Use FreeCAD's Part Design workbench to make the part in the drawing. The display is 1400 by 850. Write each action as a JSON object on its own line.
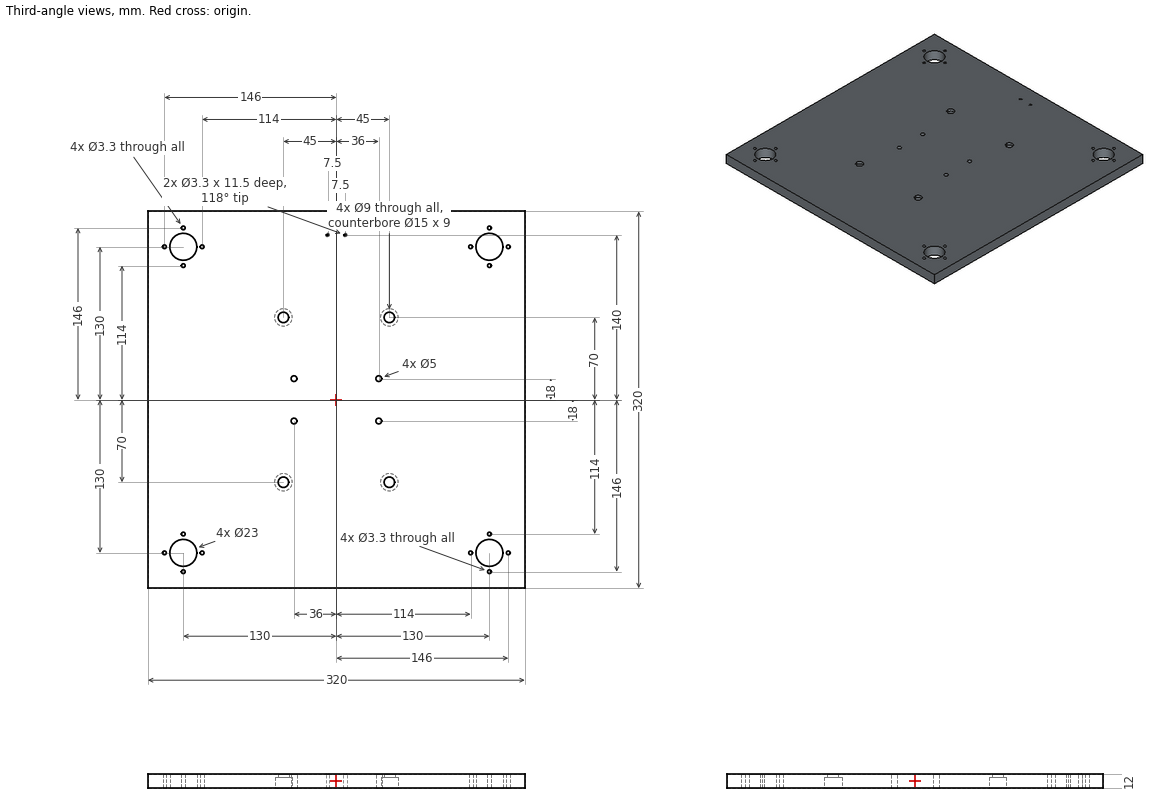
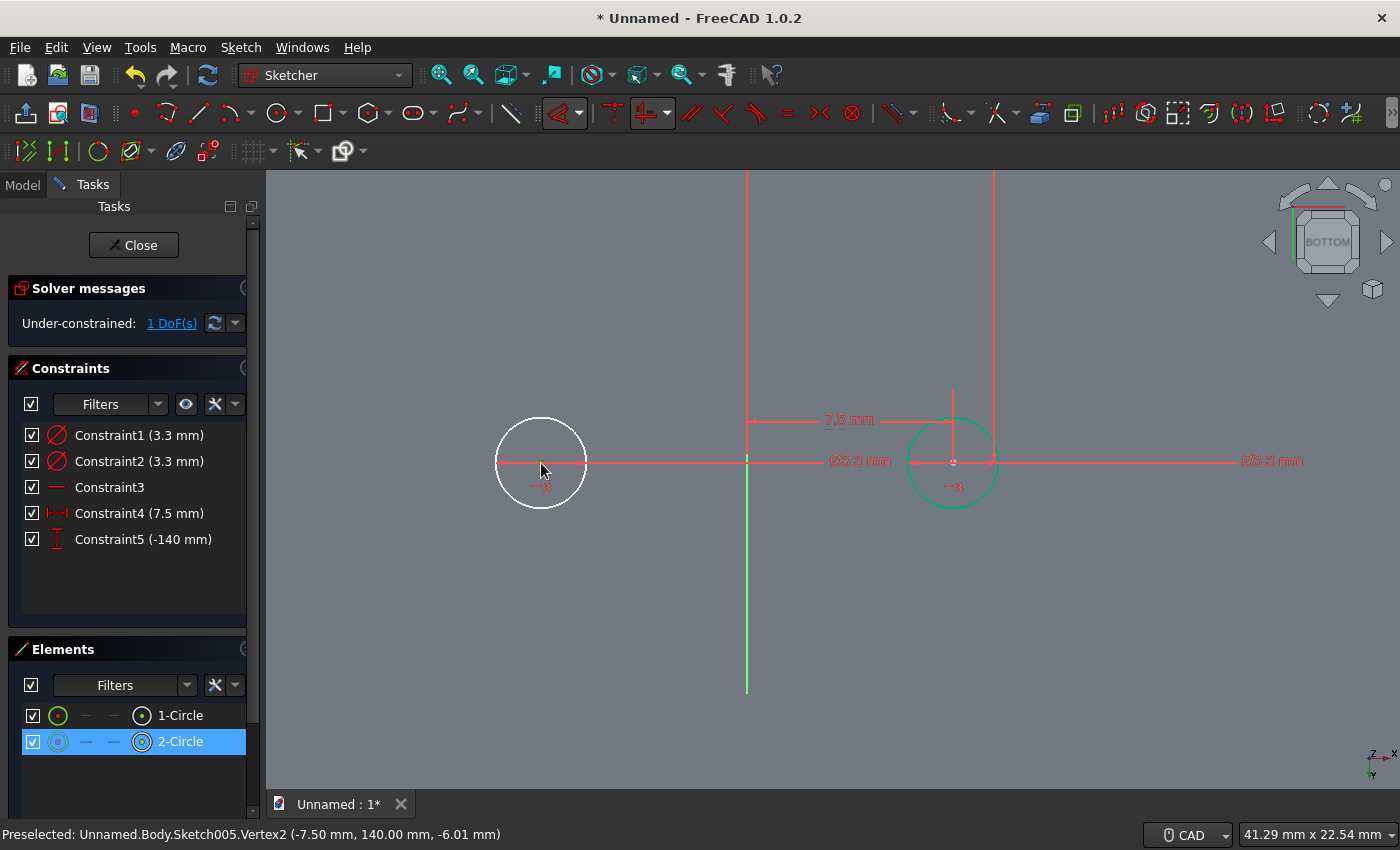
{"action": "left_click", "coordinate": [582, 114]}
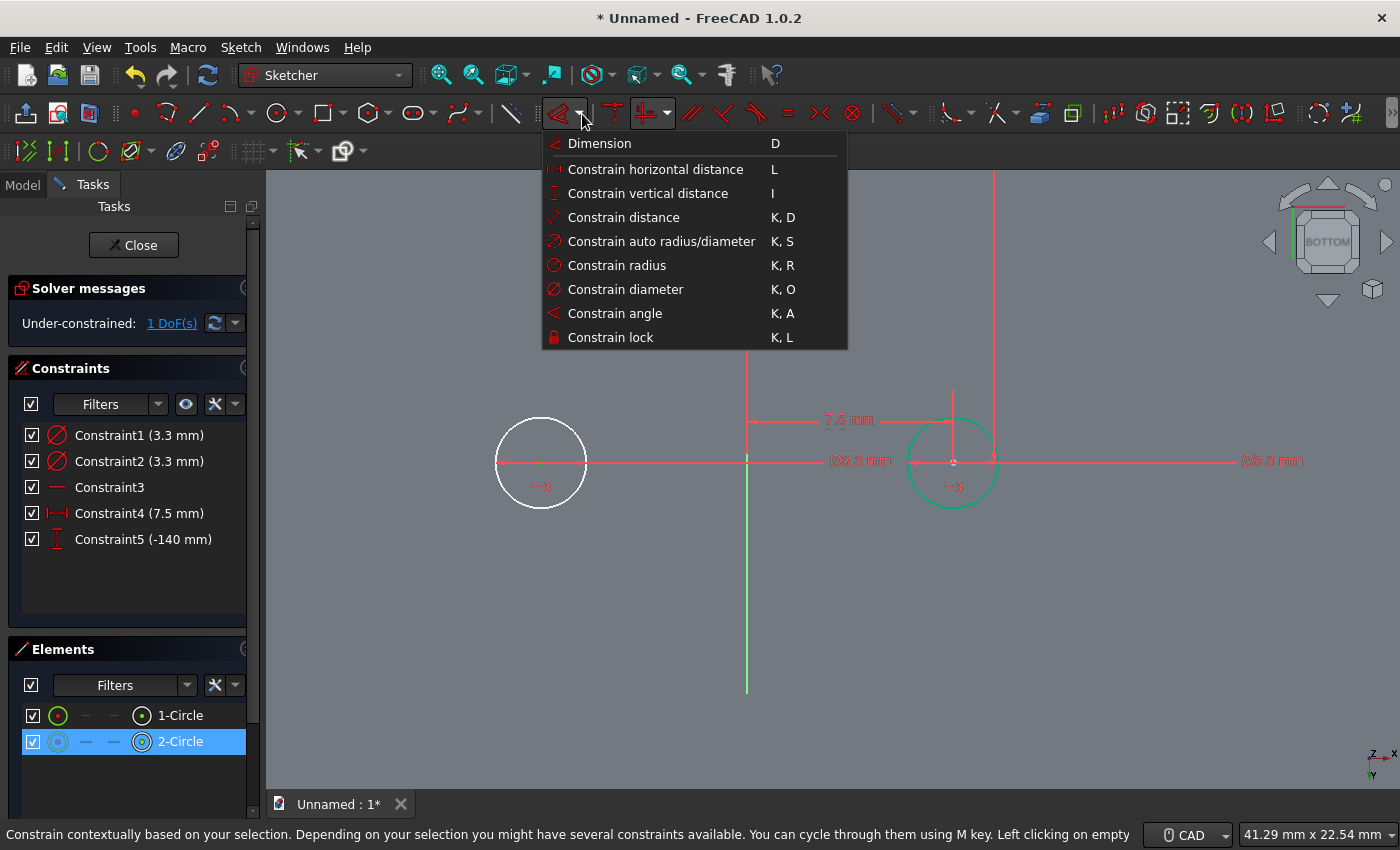
{"action": "left_click", "coordinate": [695, 169]}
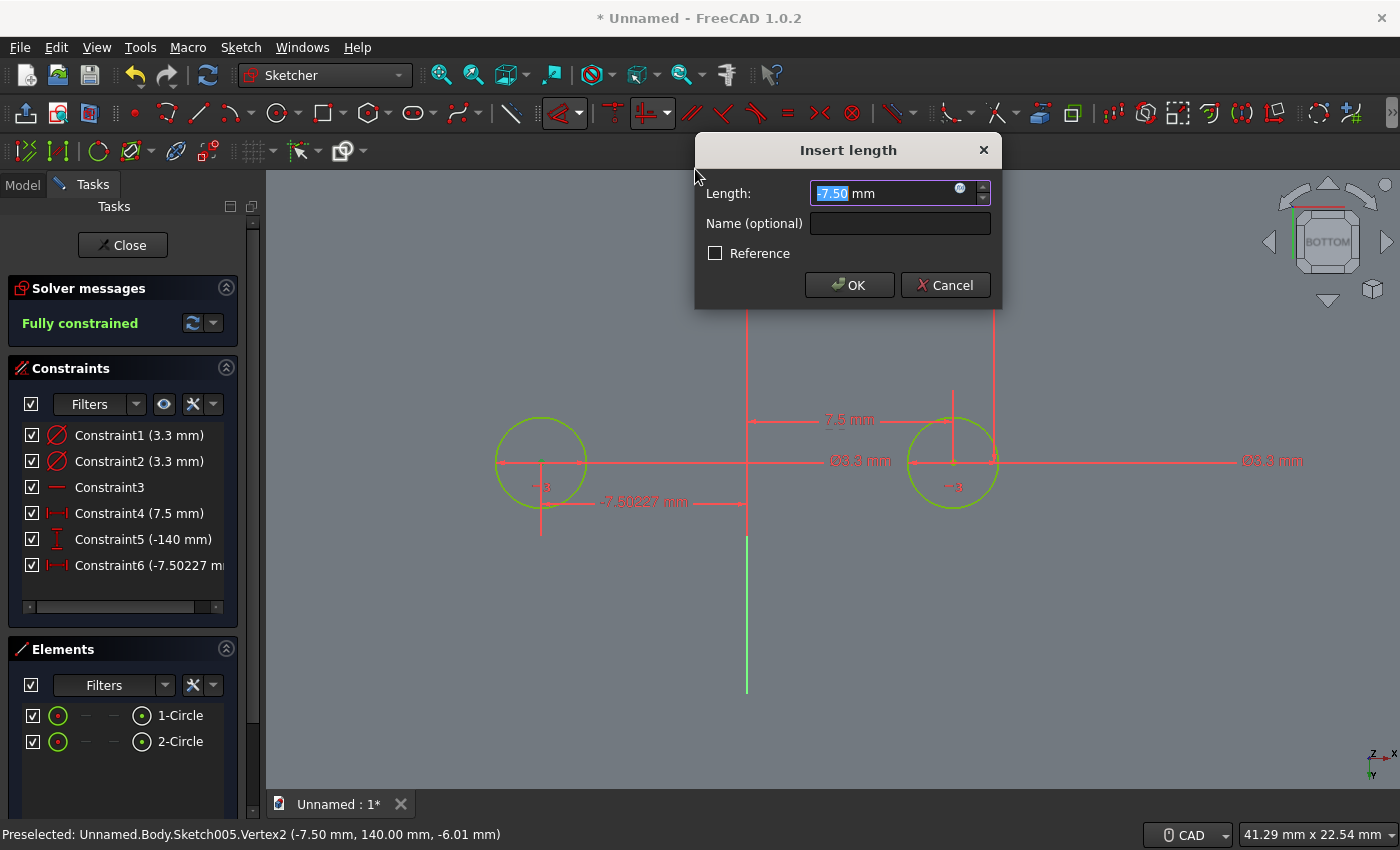
{"action": "type", "text": "-7.5"}
{"action": "key", "text": "Return"}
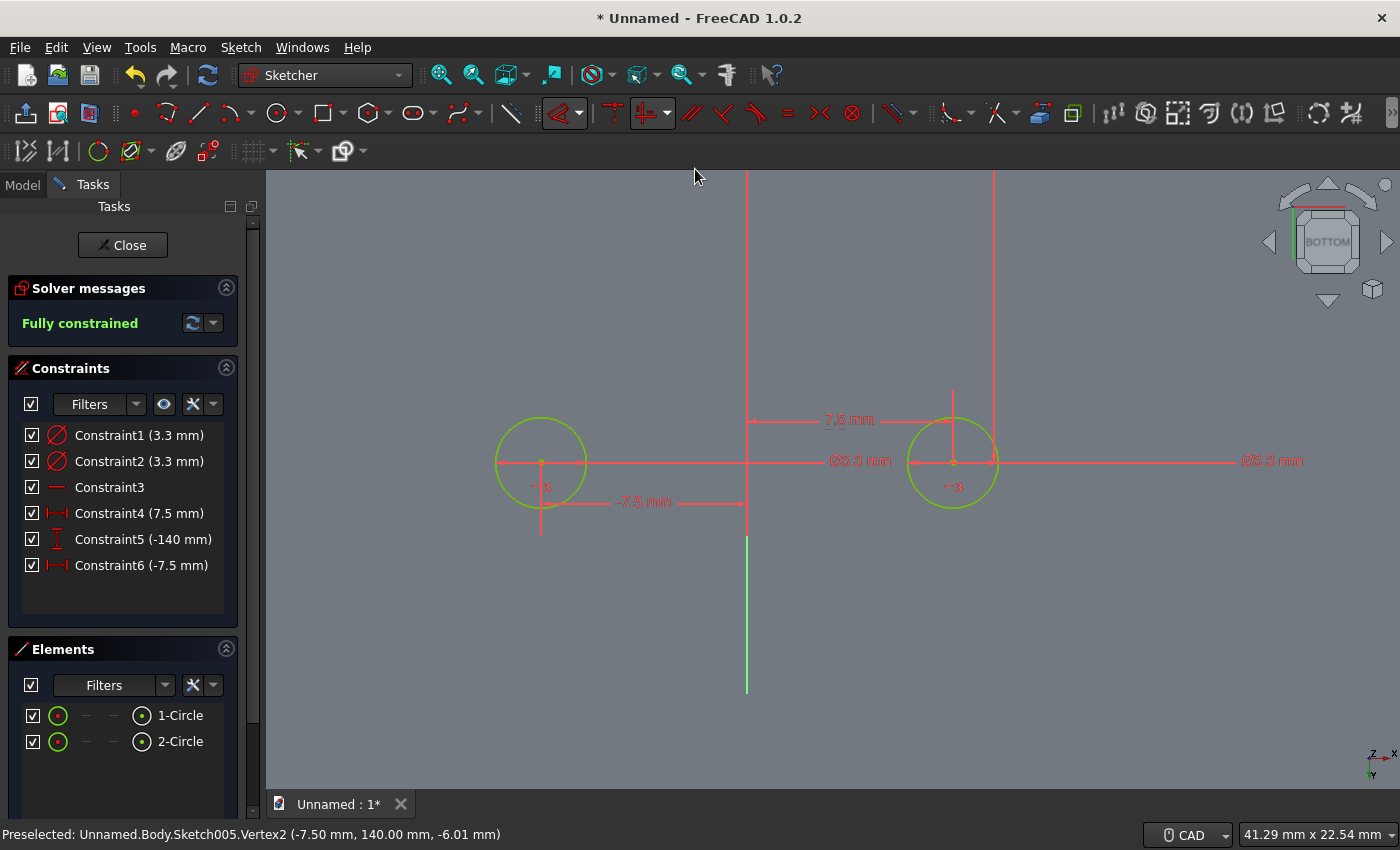
{"action": "left_click", "coordinate": [123, 245]}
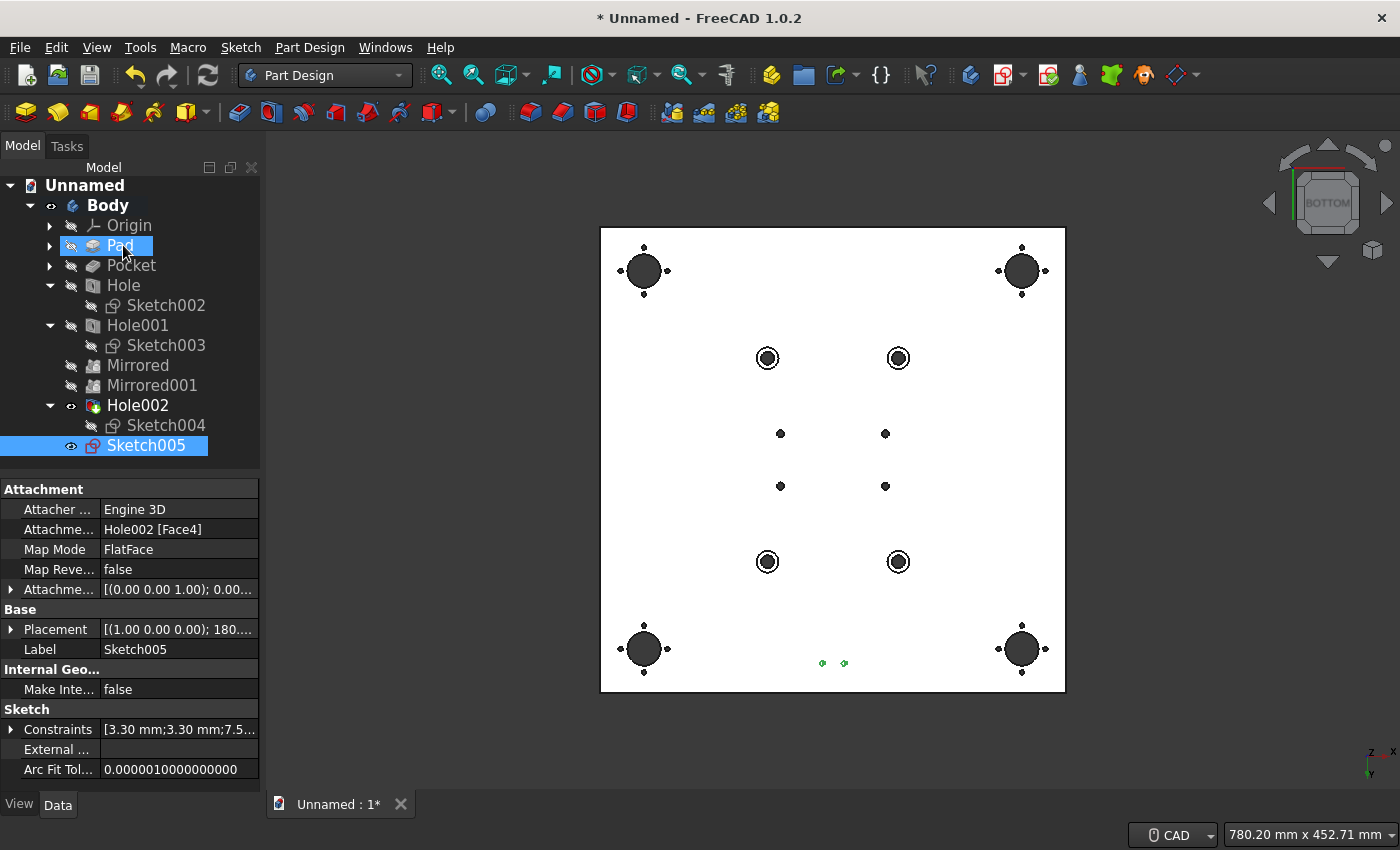
{"action": "left_click", "coordinate": [272, 112]}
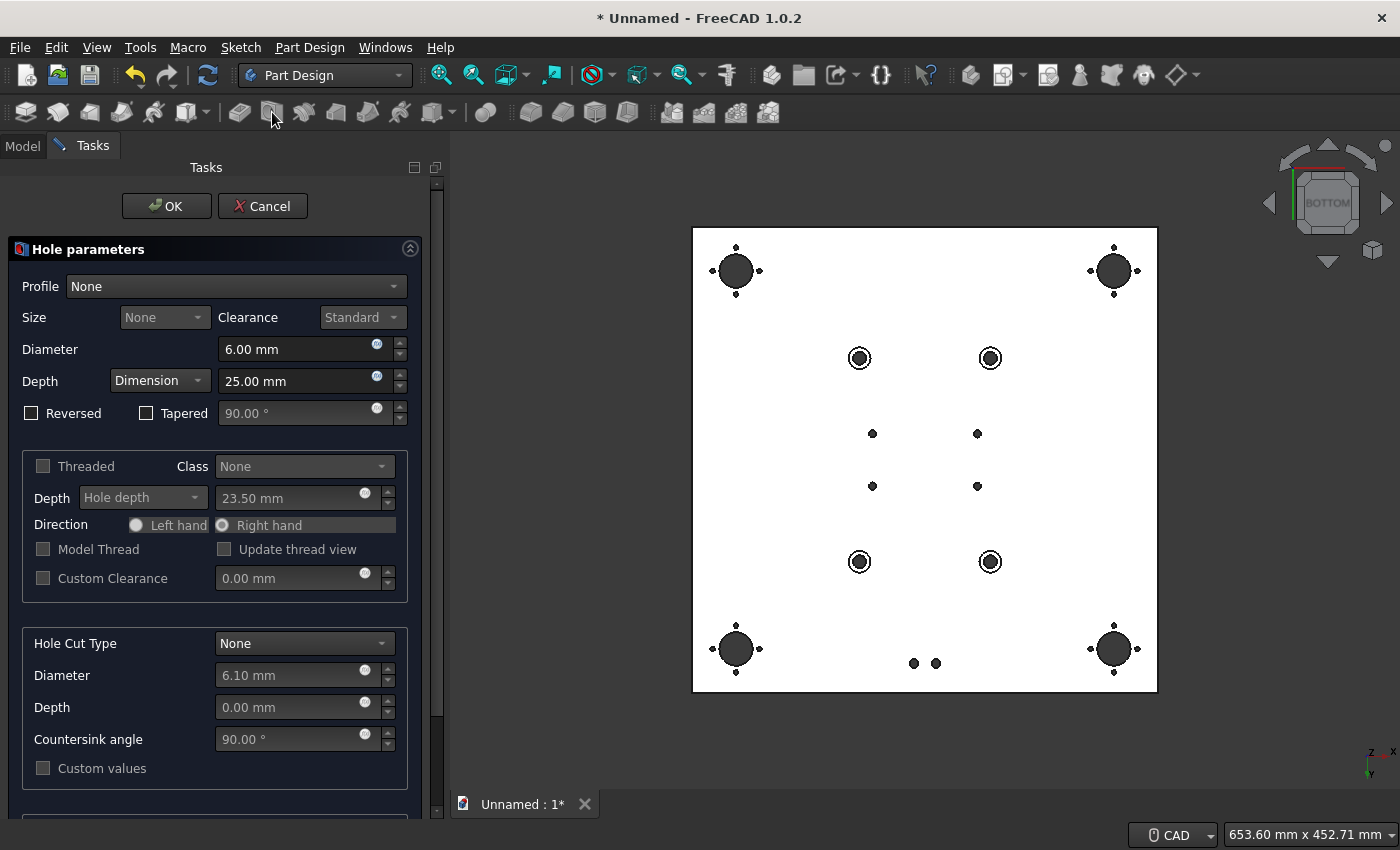
{"action": "triple_click", "coordinate": [305, 349]}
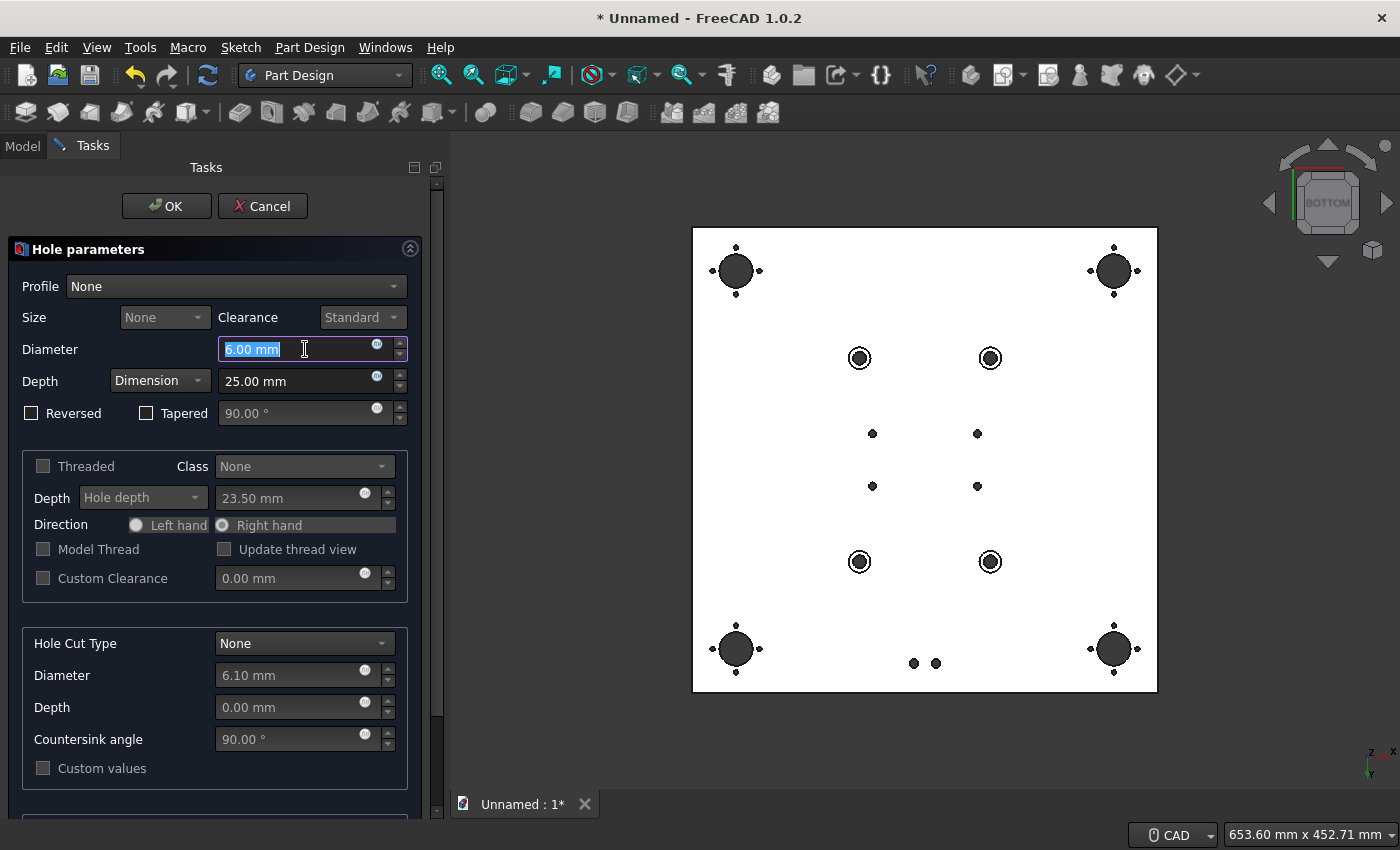
{"action": "type", "text": "3.3"}
{"action": "key", "text": "Tab"}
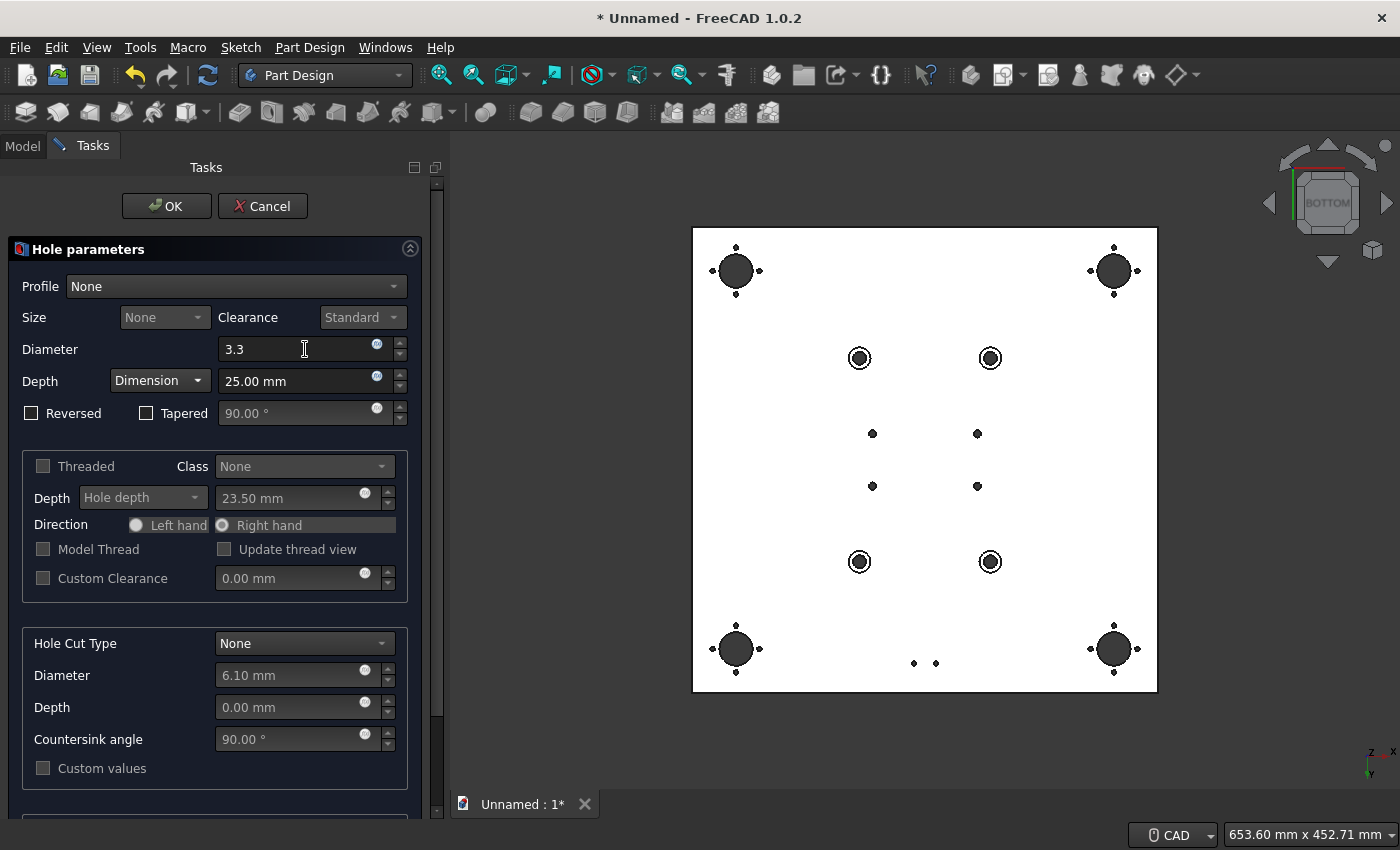
{"action": "triple_click", "coordinate": [305, 381]}